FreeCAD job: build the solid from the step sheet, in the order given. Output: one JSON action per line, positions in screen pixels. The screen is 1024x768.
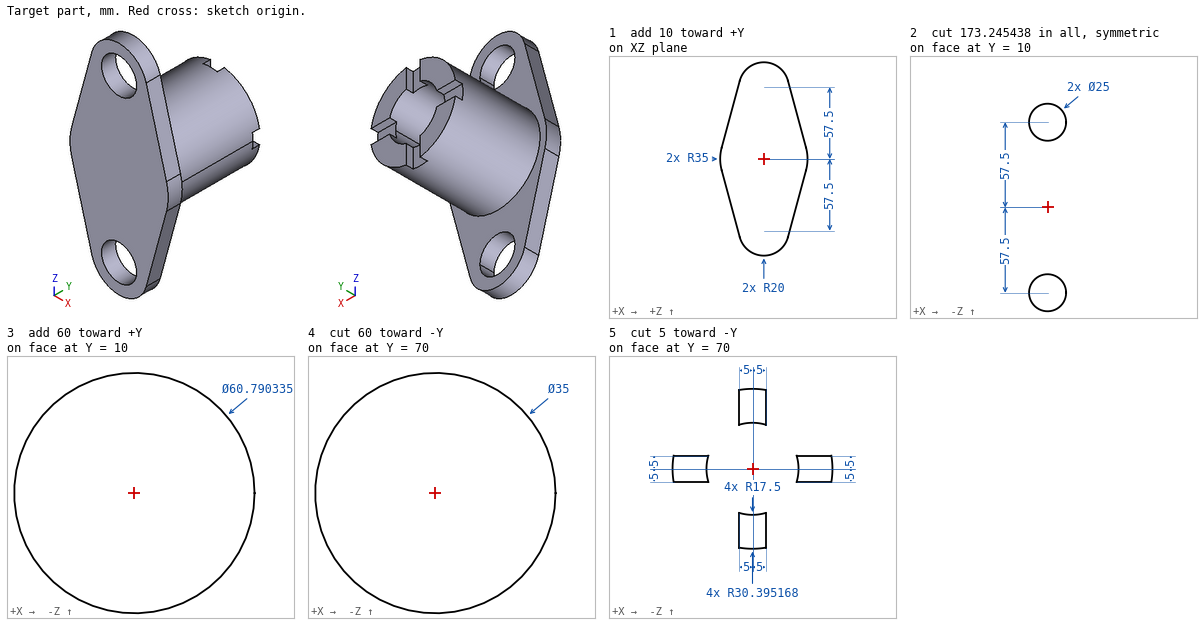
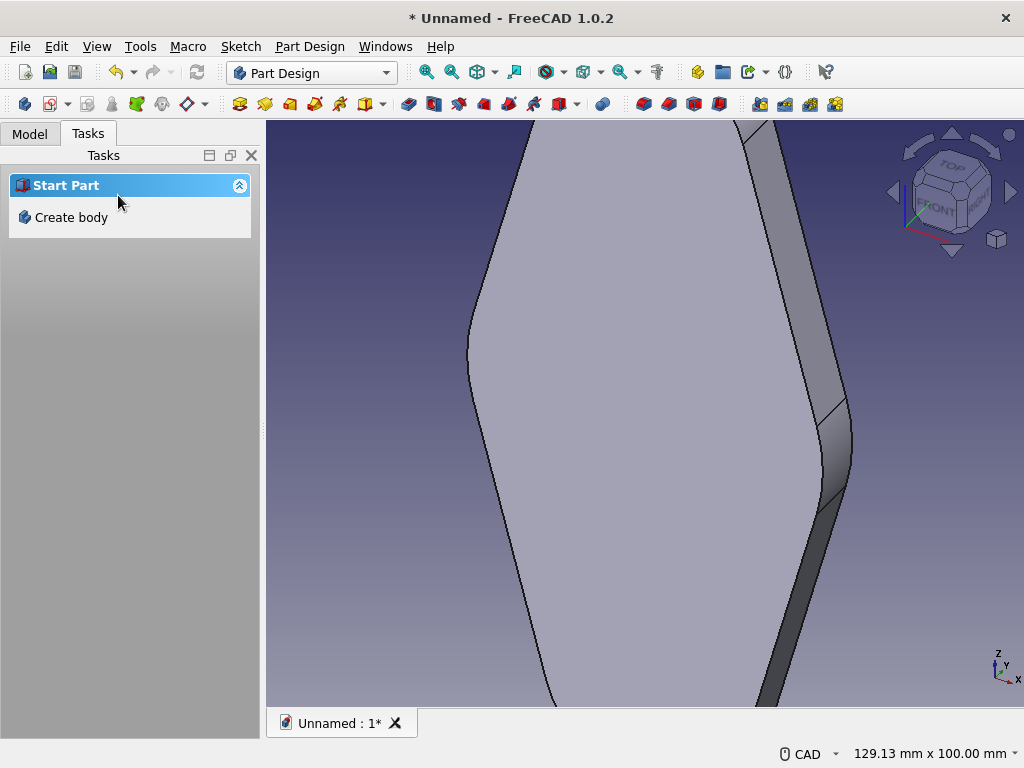
{"action": "left_click", "coordinate": [427, 72]}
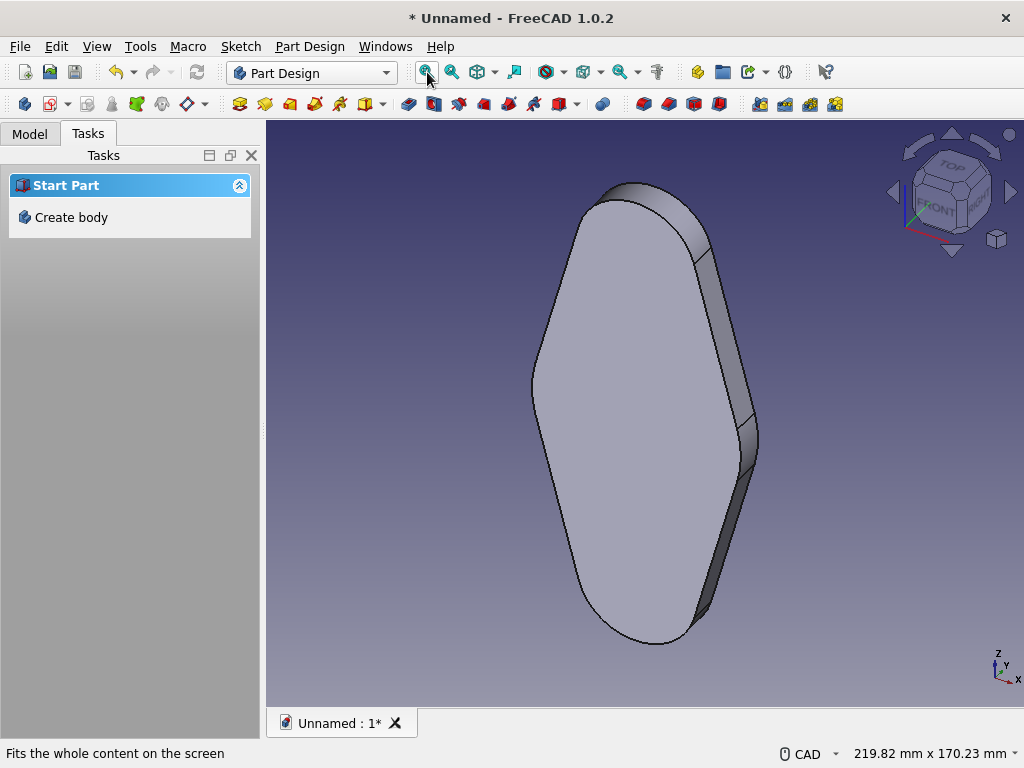
{"action": "key", "text": "4"}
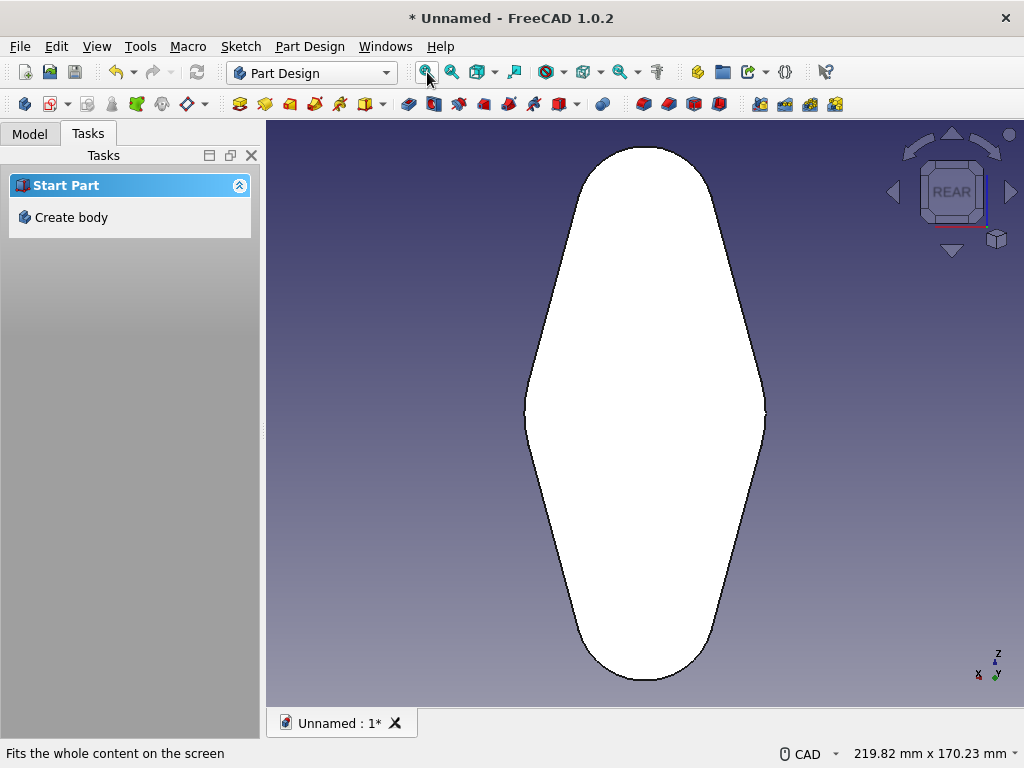
{"action": "left_click", "coordinate": [645, 412]}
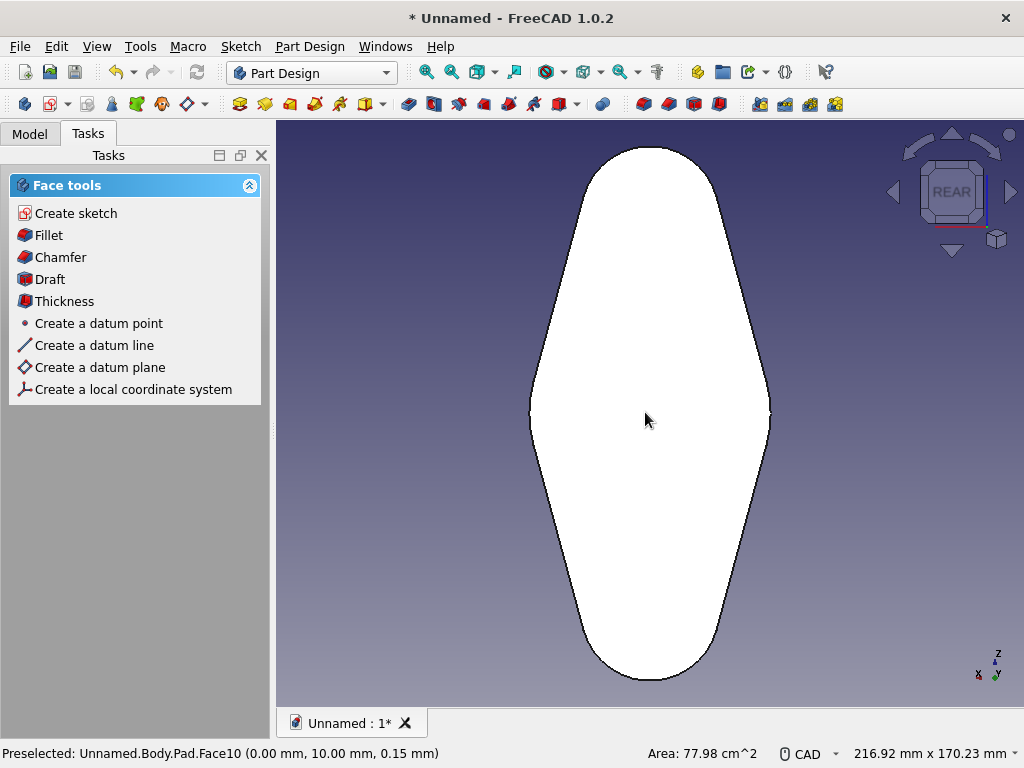
{"action": "left_click", "coordinate": [50, 104]}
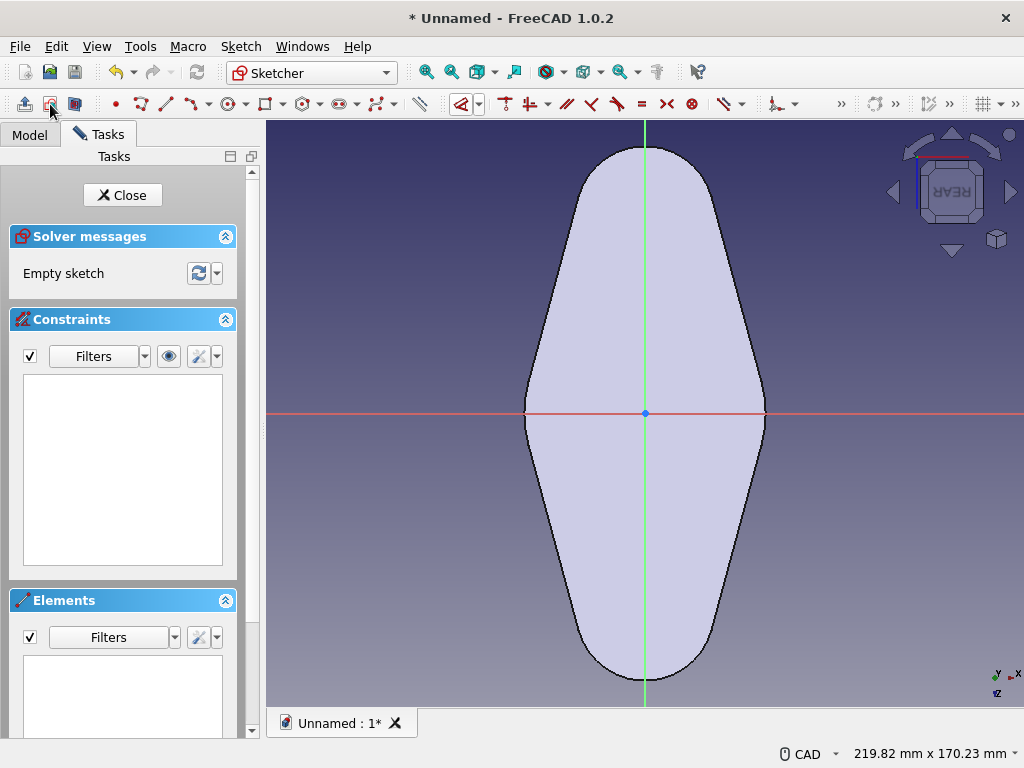
{"action": "scroll", "coordinate": [294, 413], "scroll_direction": "down", "scroll_amount": 1}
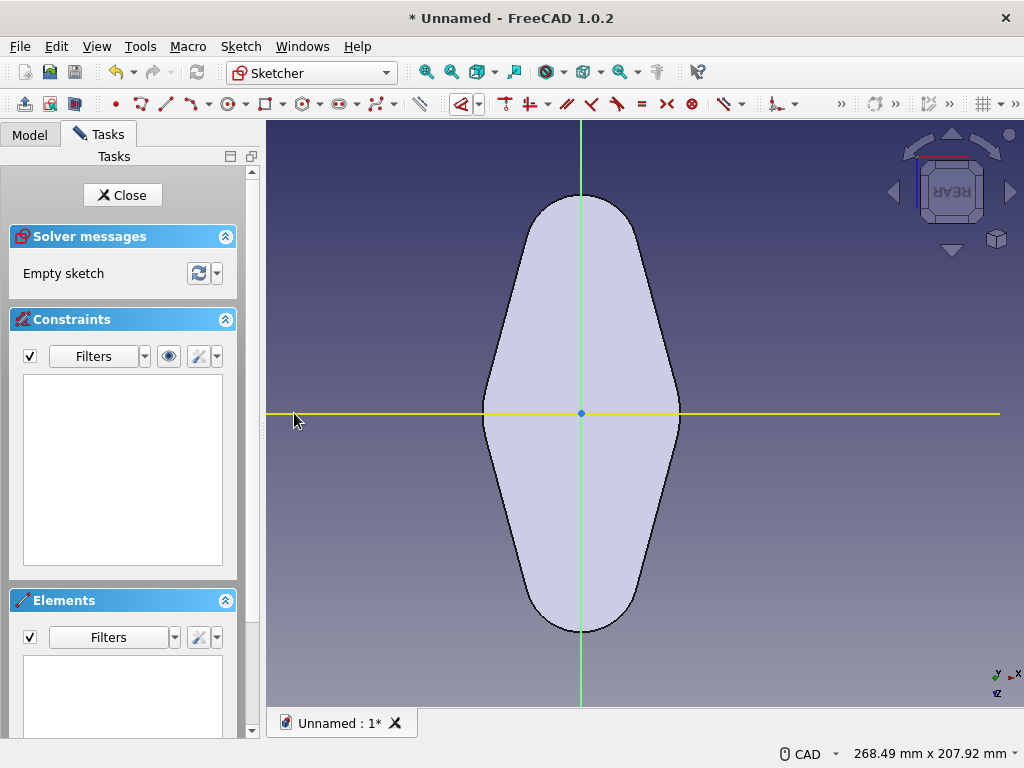
{"action": "key", "text": "g c"}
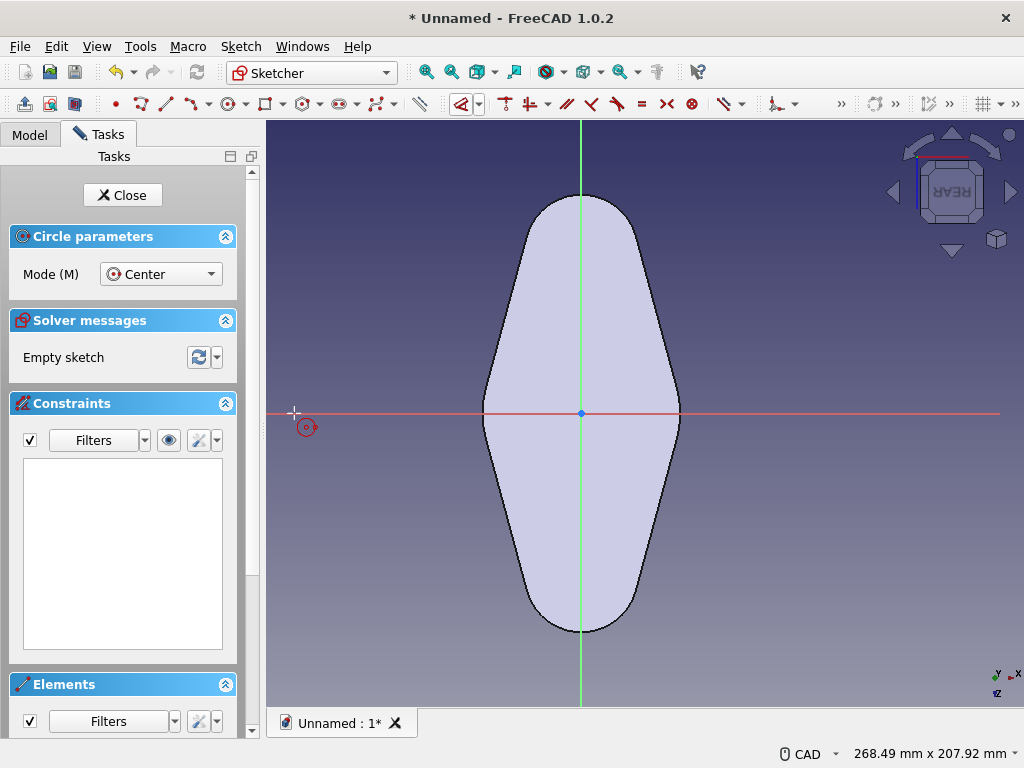
{"action": "left_click", "coordinate": [581, 251]}
{"action": "mouse_move", "coordinate": [606, 226]}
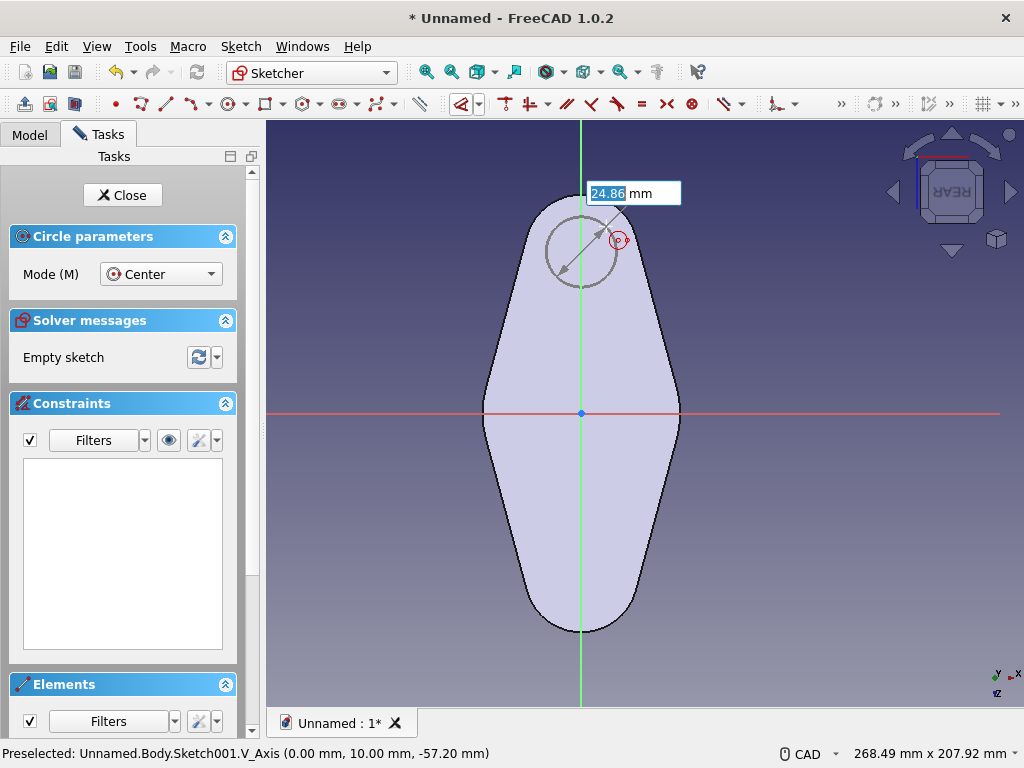
{"action": "type", "text": "25"}
{"action": "key", "text": "Return"}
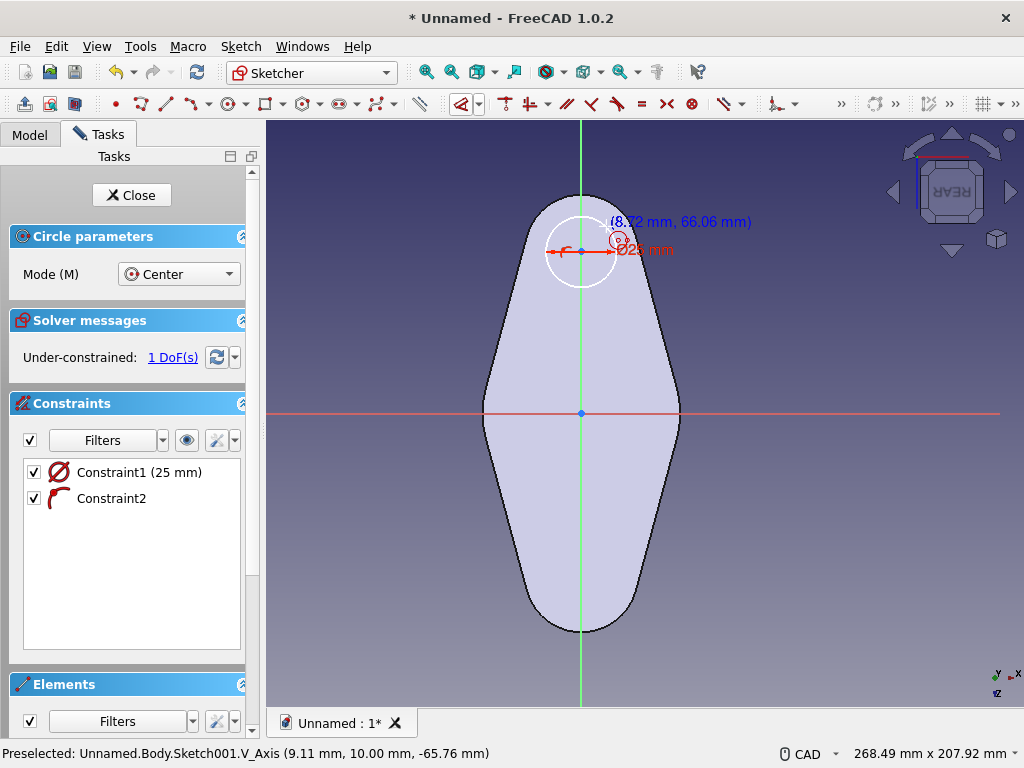
{"action": "left_click", "coordinate": [581, 576]}
{"action": "mouse_move", "coordinate": [606, 551]}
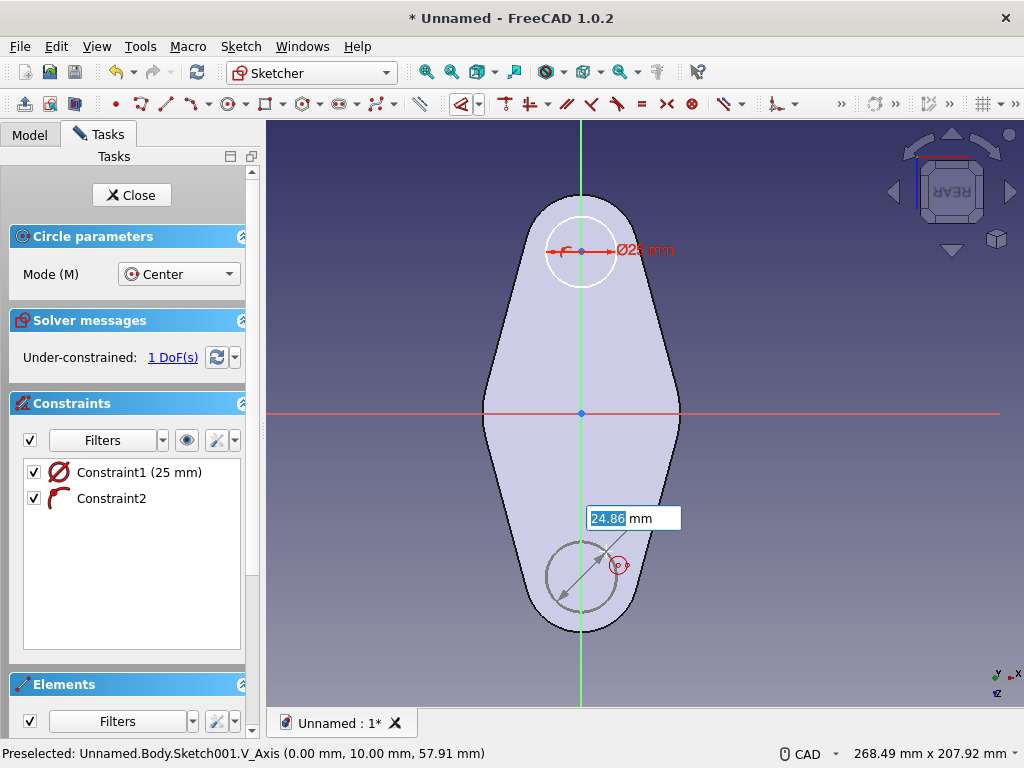
{"action": "type", "text": "25"}
{"action": "key", "text": "Return"}
{"action": "key", "text": "Escape"}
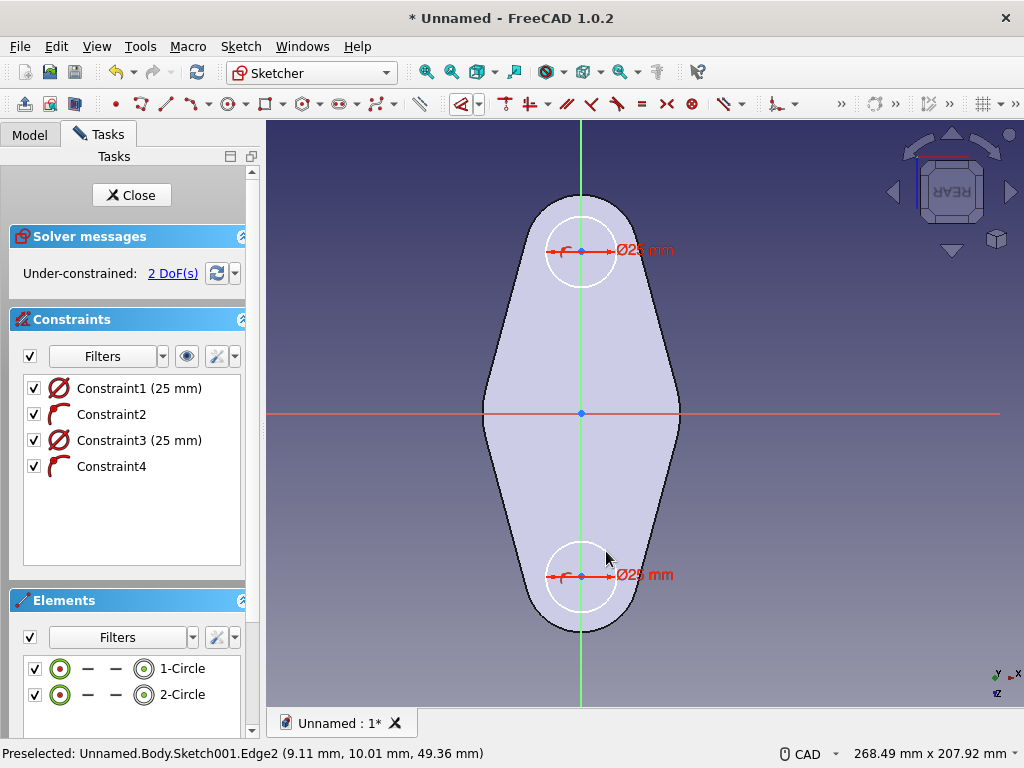
{"action": "left_click", "coordinate": [581, 252]}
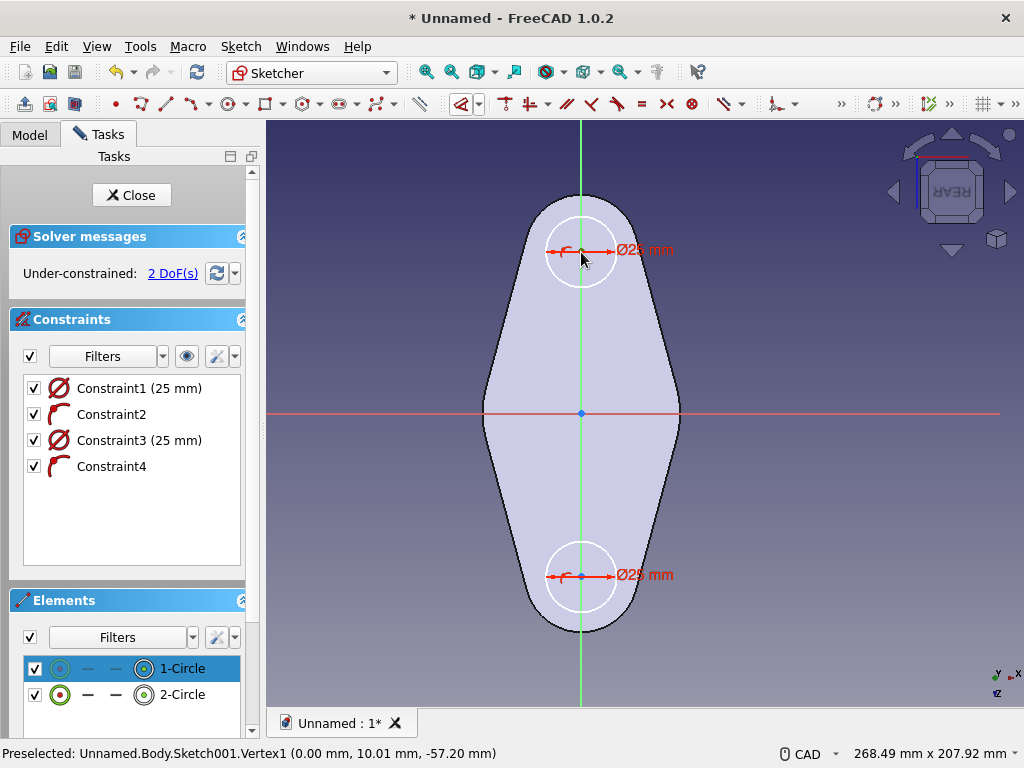
{"action": "left_click", "coordinate": [478, 104]}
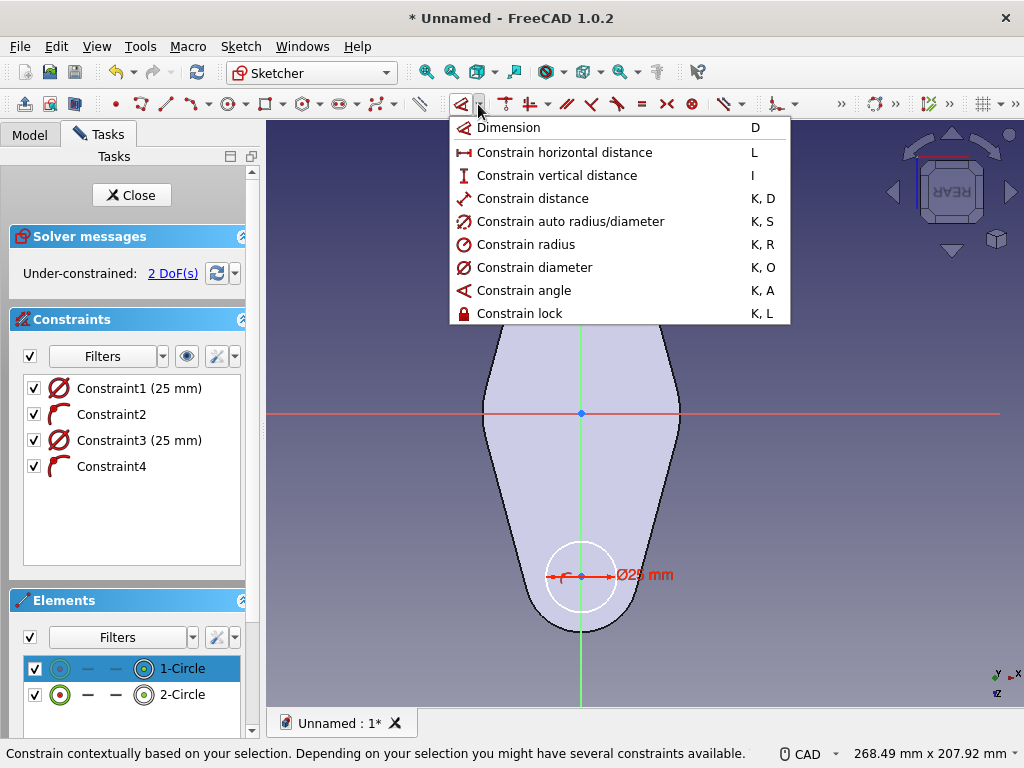
{"action": "left_click", "coordinate": [620, 176]}